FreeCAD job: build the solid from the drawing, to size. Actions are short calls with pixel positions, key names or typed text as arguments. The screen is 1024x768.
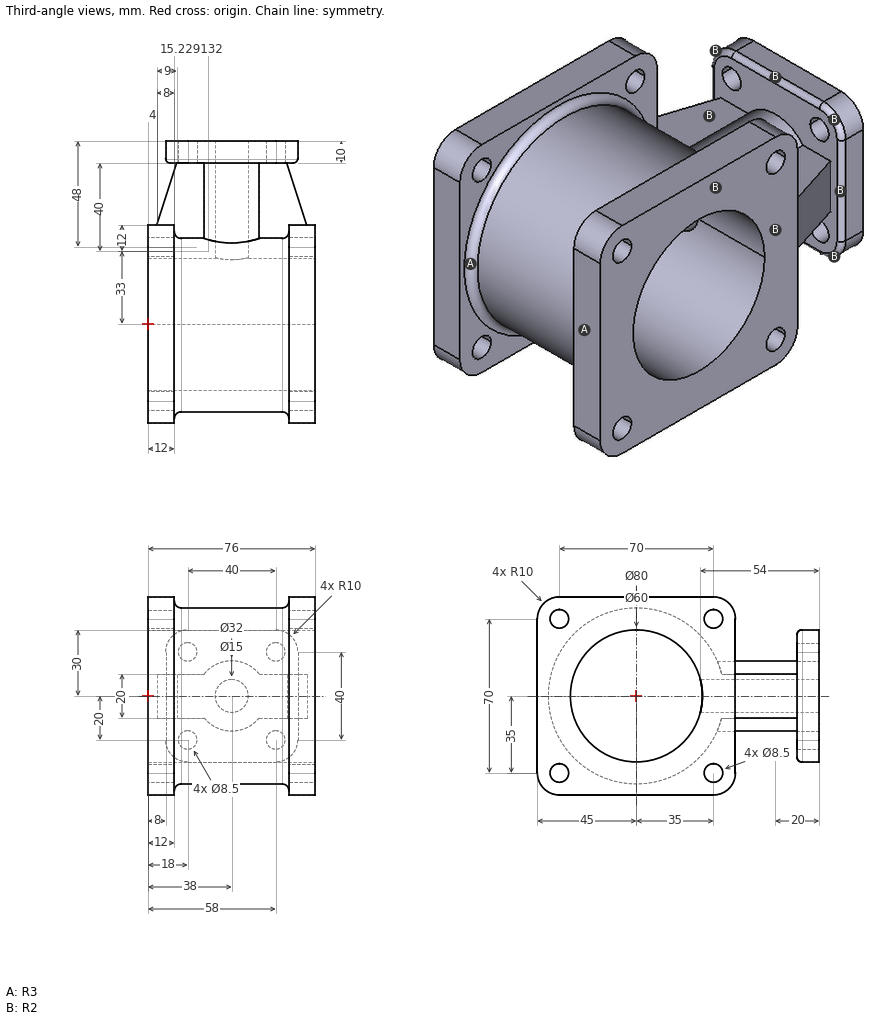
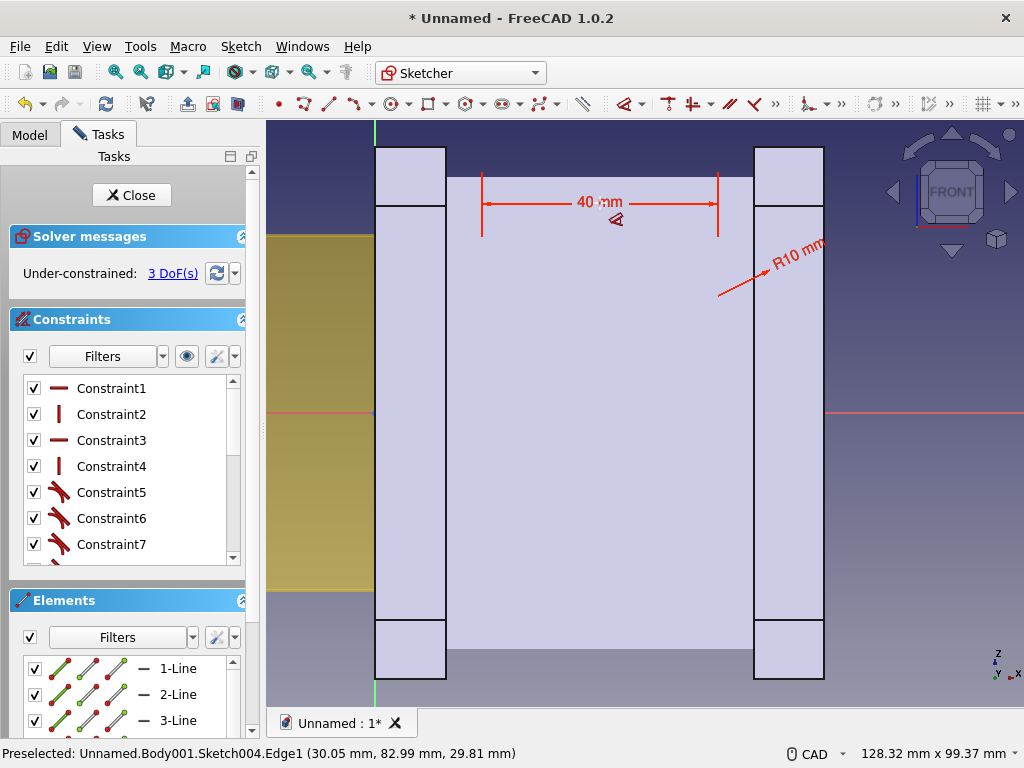
click(777, 367)
click(811, 360)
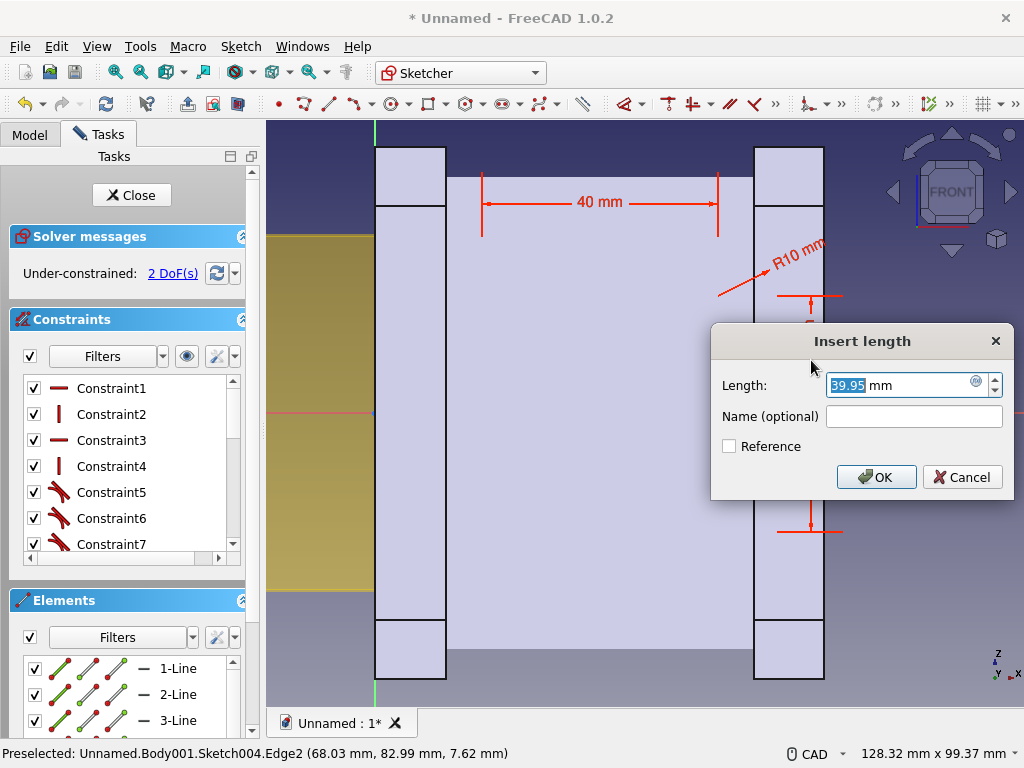
text(40)
key(Return)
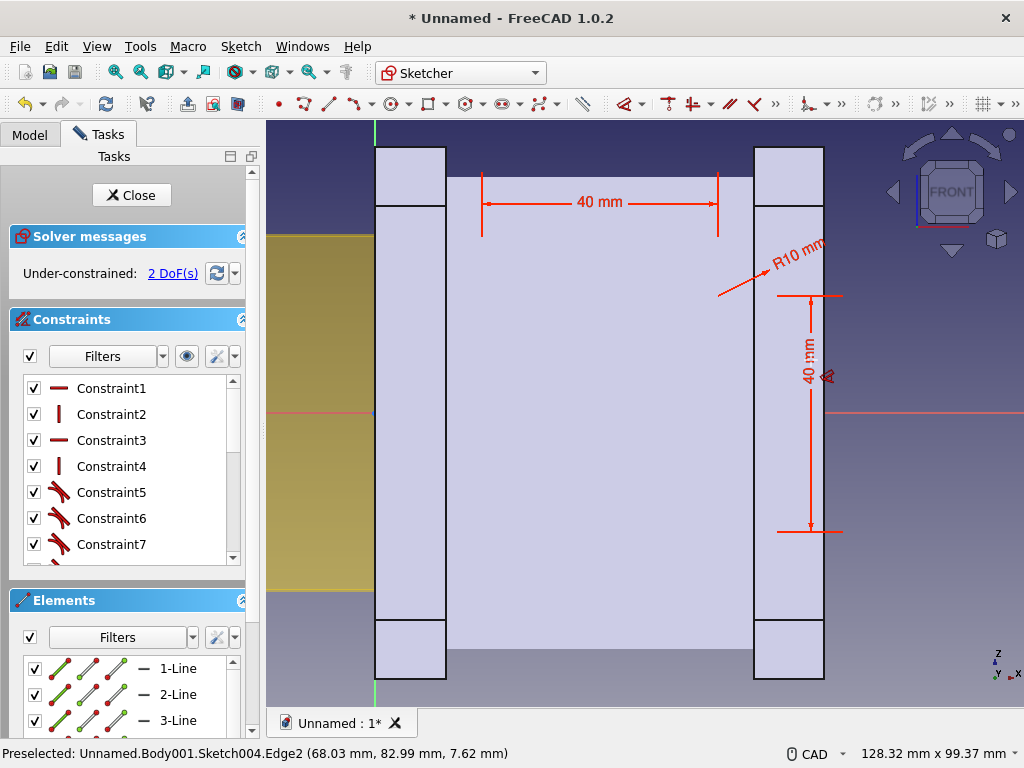
click(423, 532)
click(399, 566)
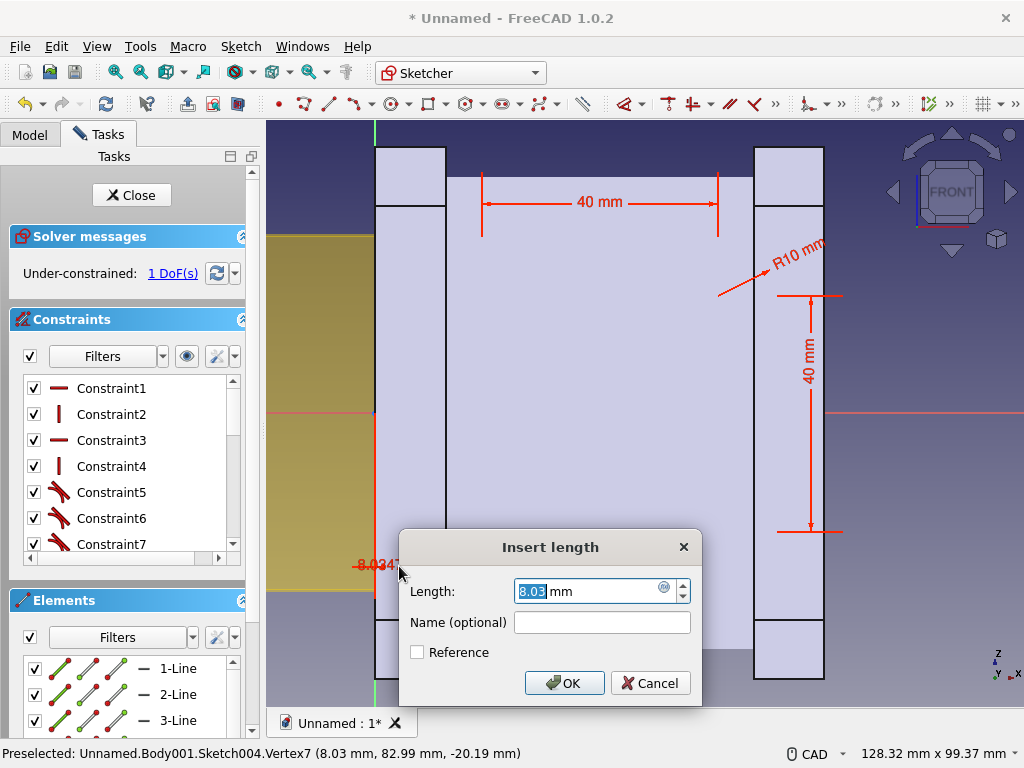
text(8)
key(Return)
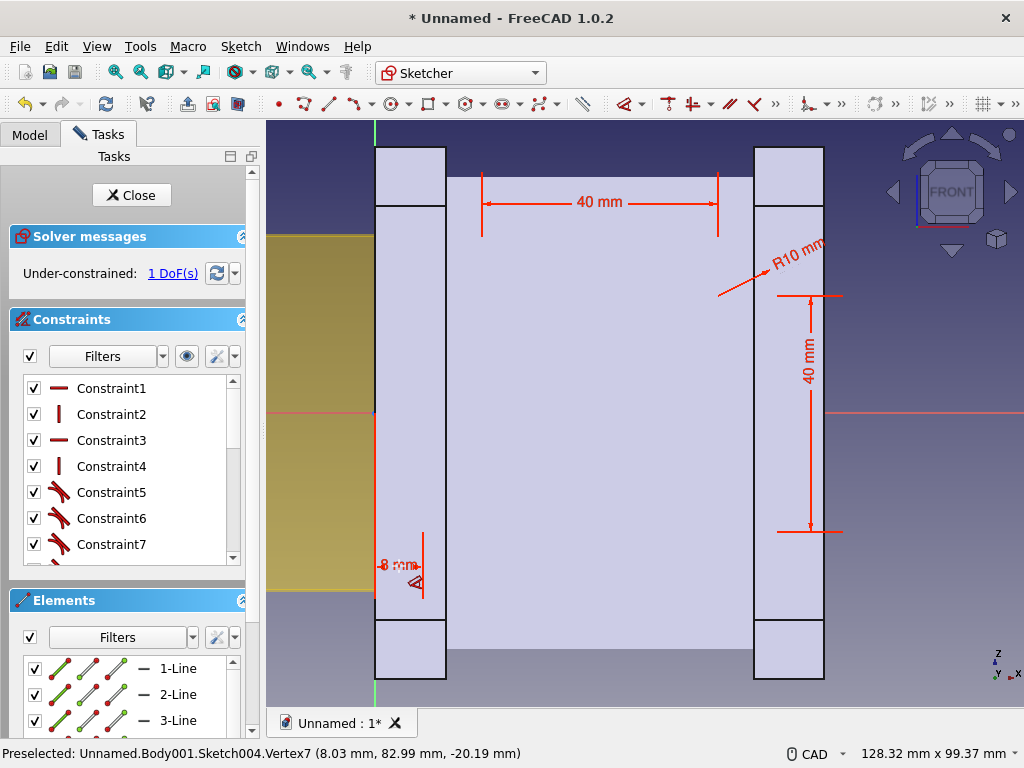
click(482, 237)
click(341, 325)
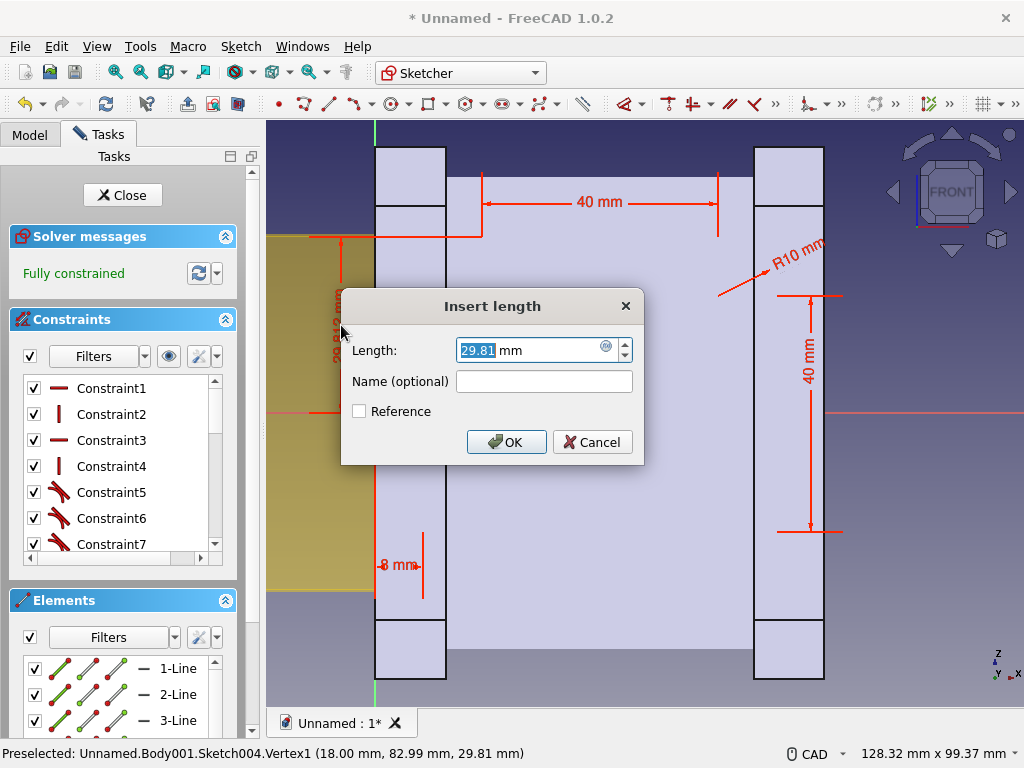
text(30)
key(Return)
key(Escape)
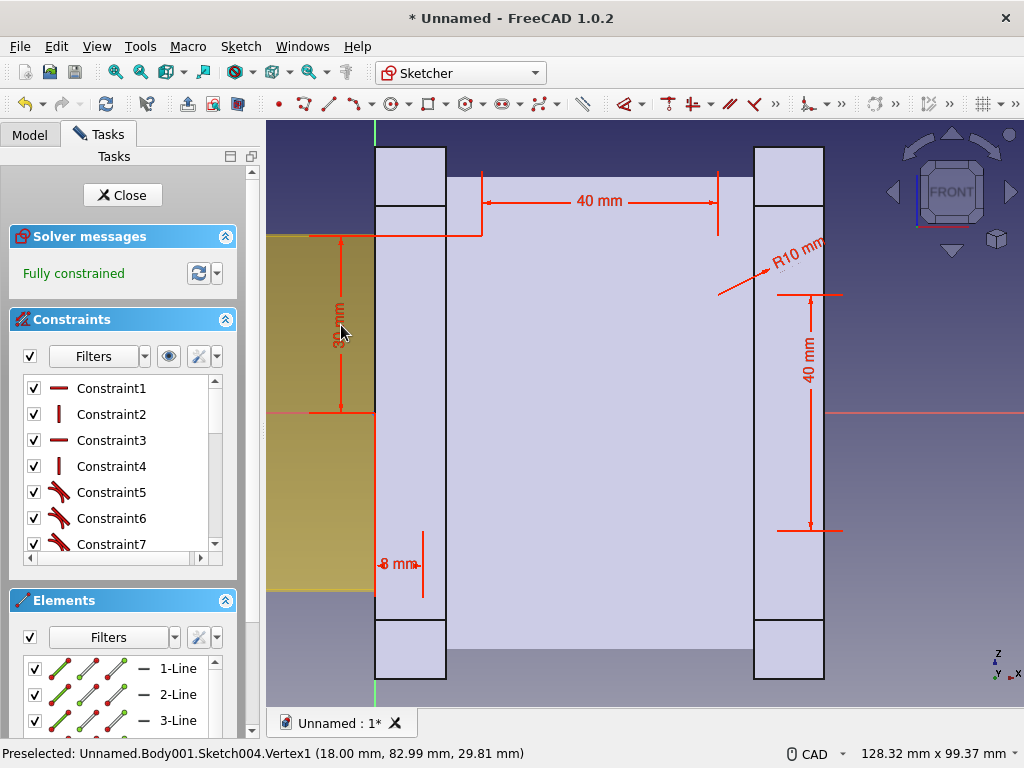
click(123, 195)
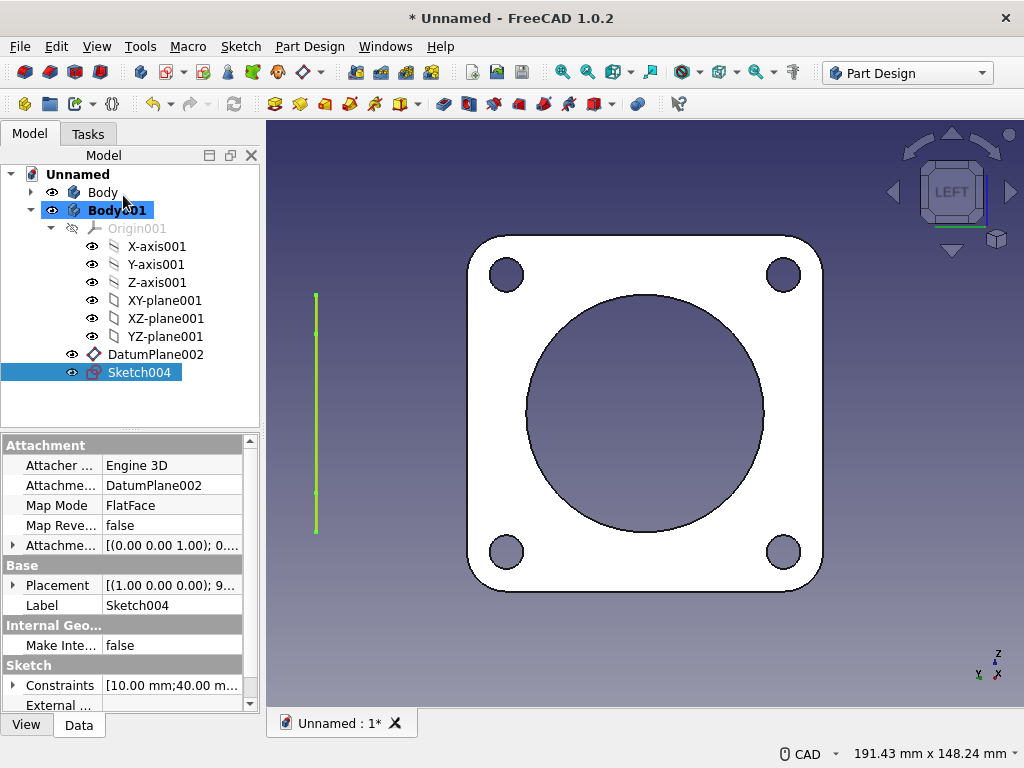
click(275, 104)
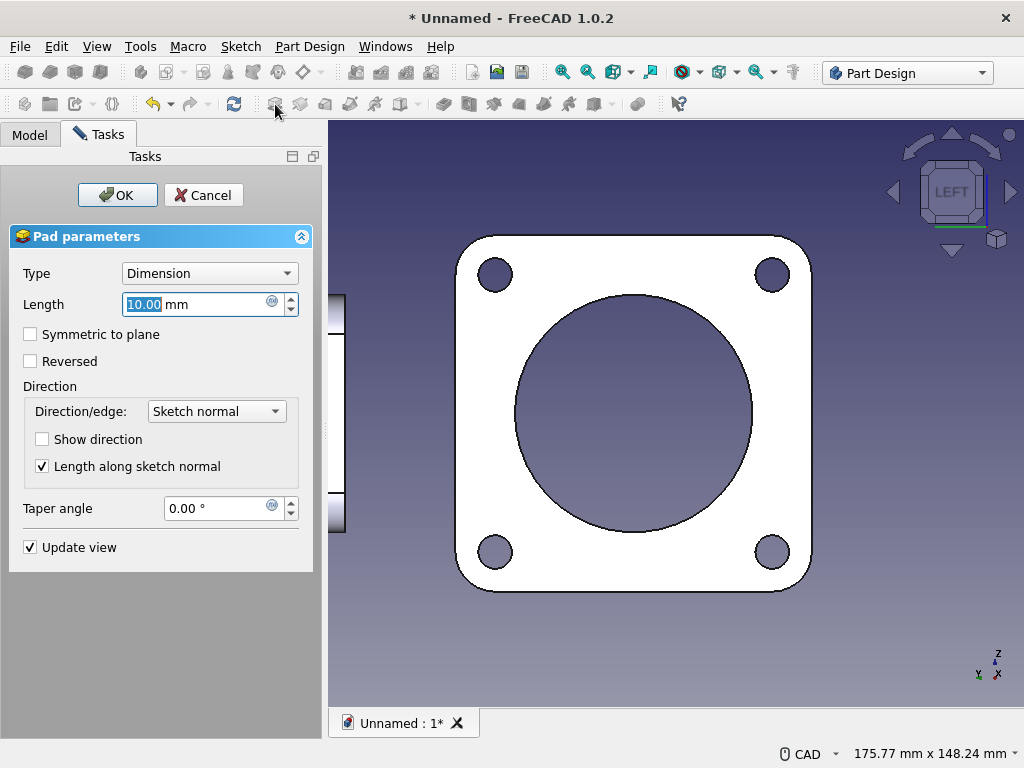
text(10)
key(Tab)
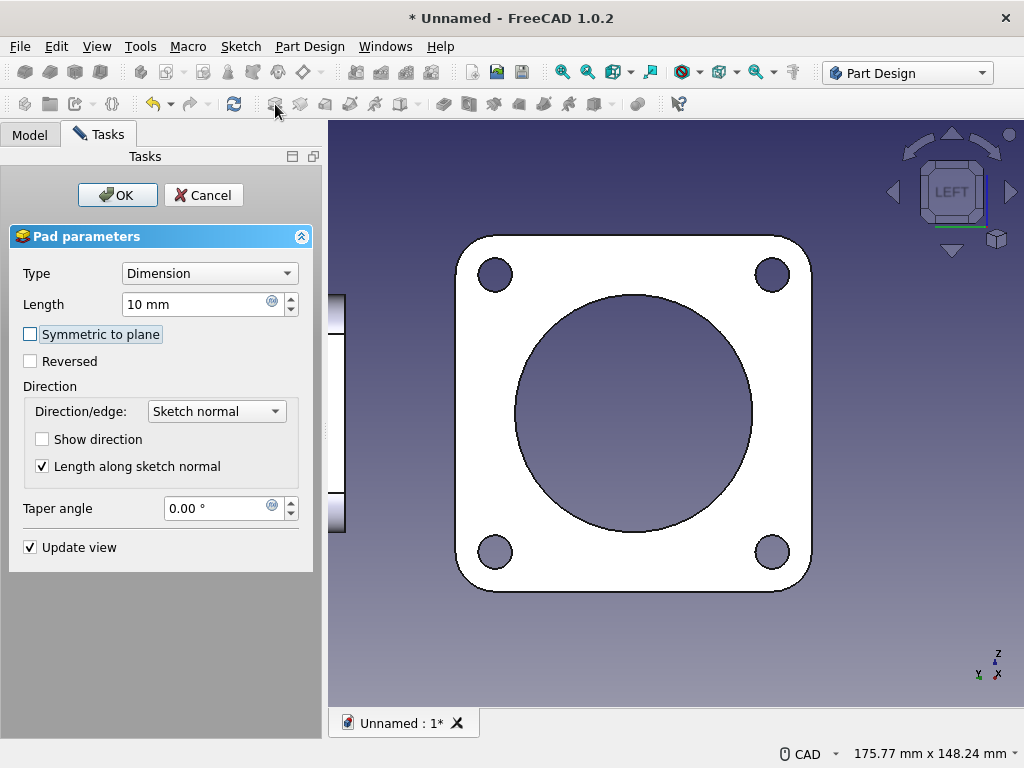
click(118, 195)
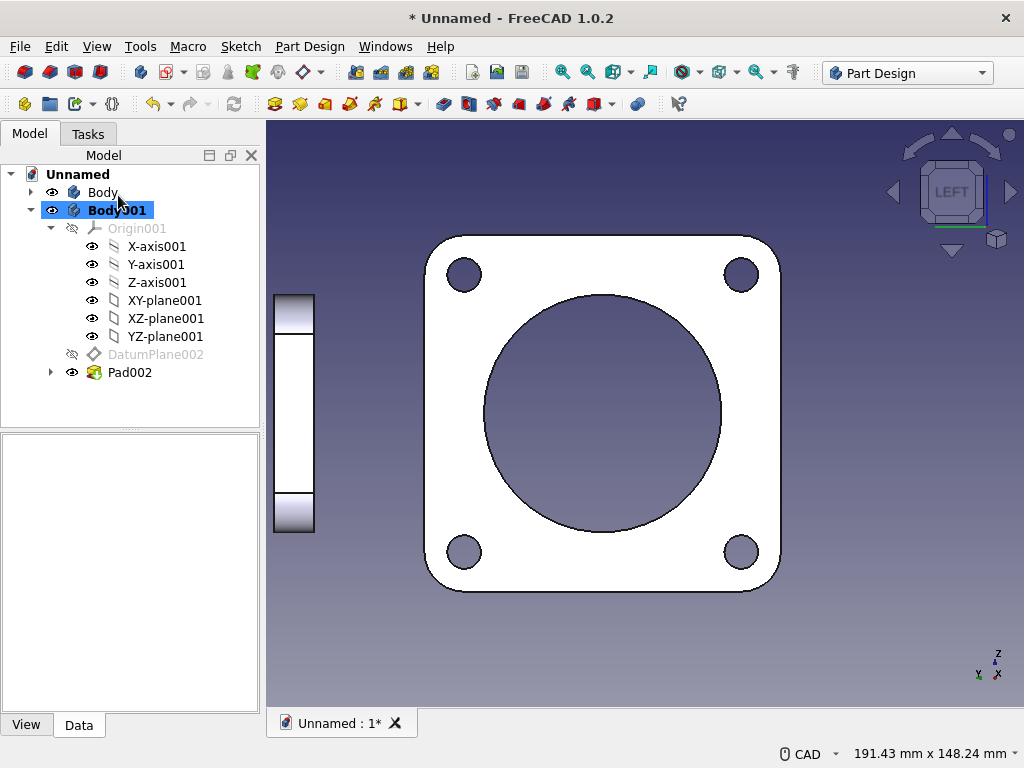
key(v)
key(f)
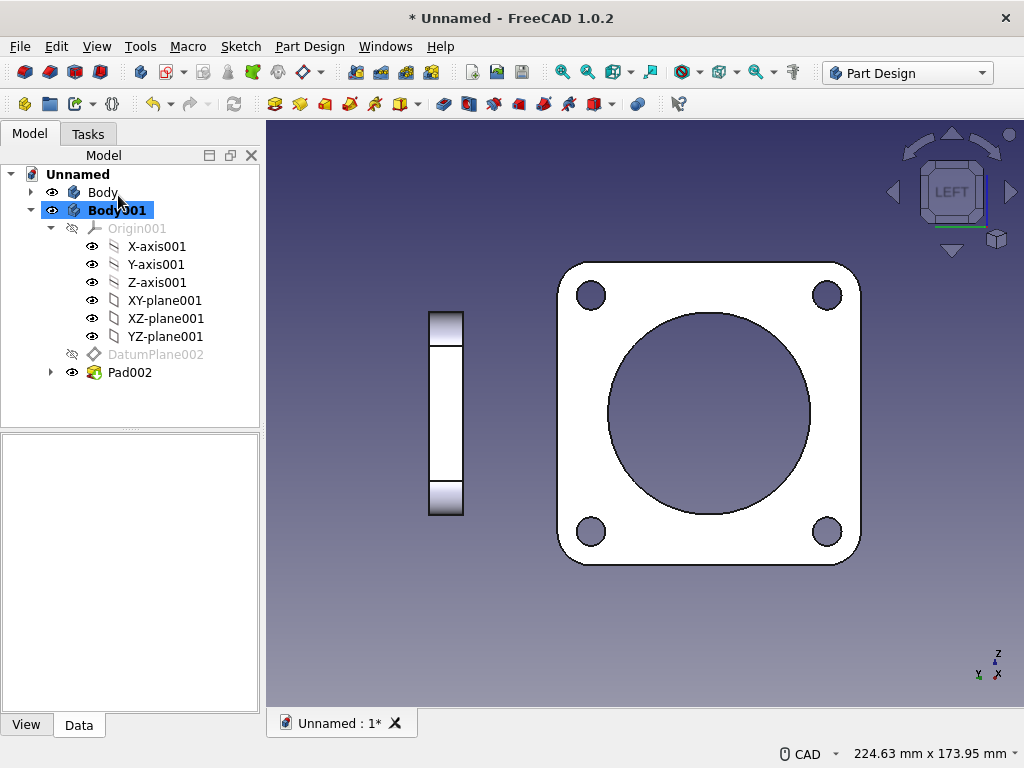
double_click(97, 192)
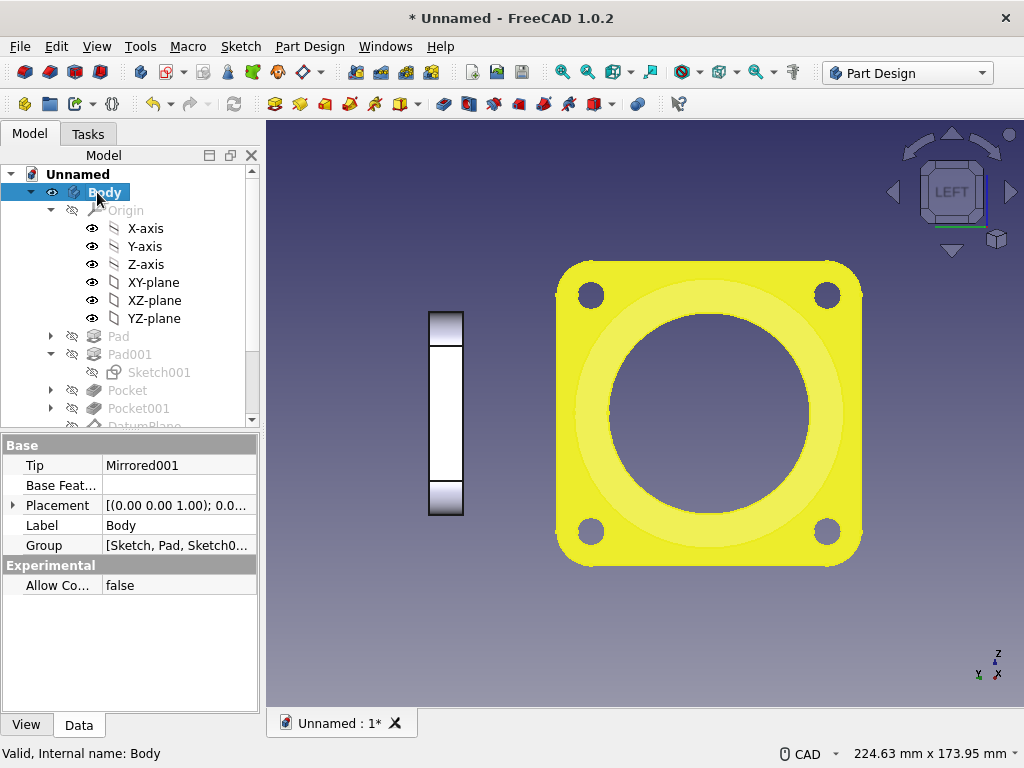
click(97, 192)